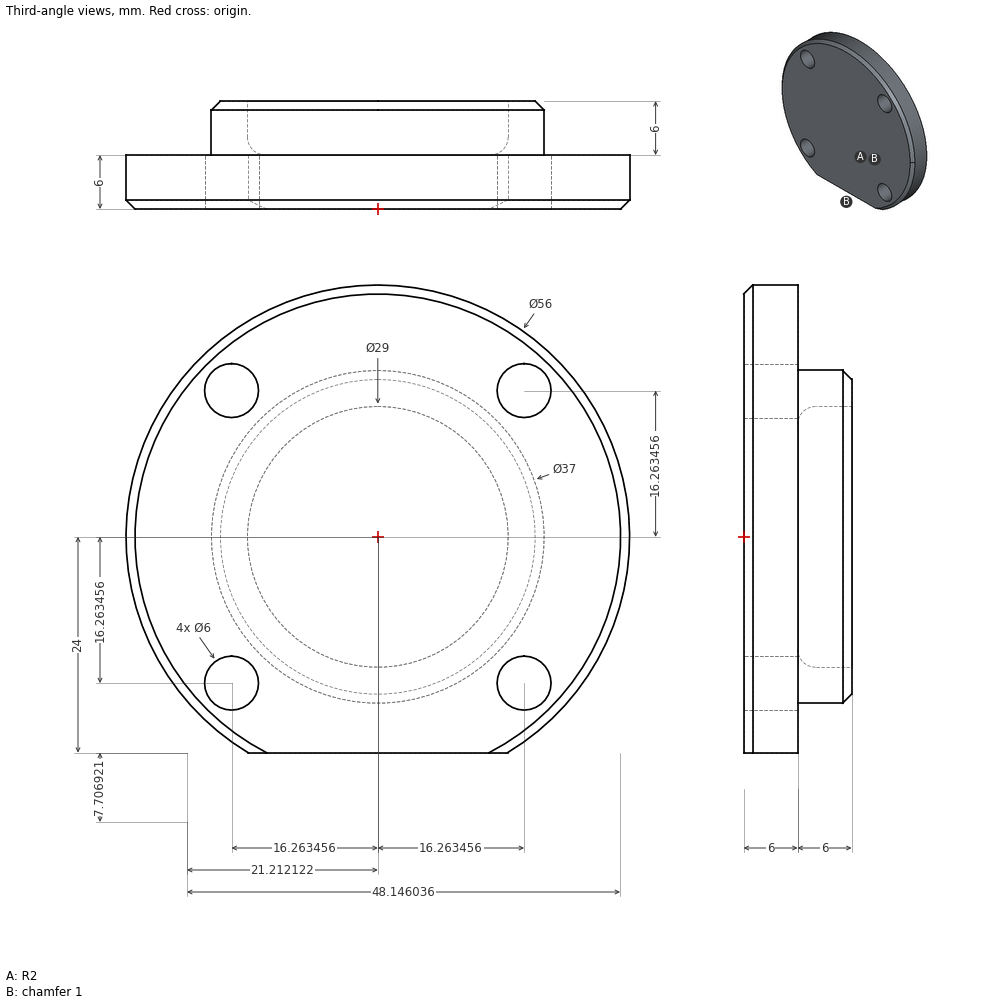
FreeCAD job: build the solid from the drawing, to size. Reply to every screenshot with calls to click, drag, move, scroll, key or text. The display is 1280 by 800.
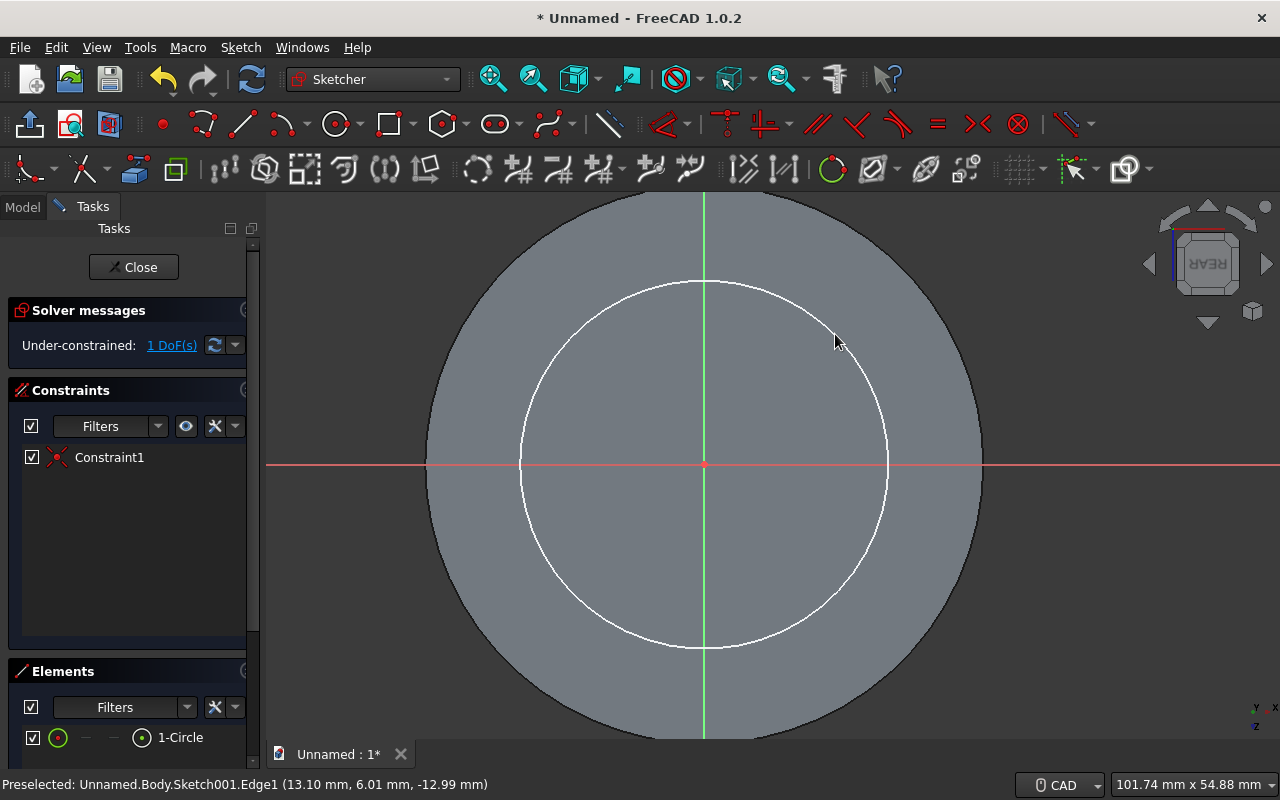
click(664, 124)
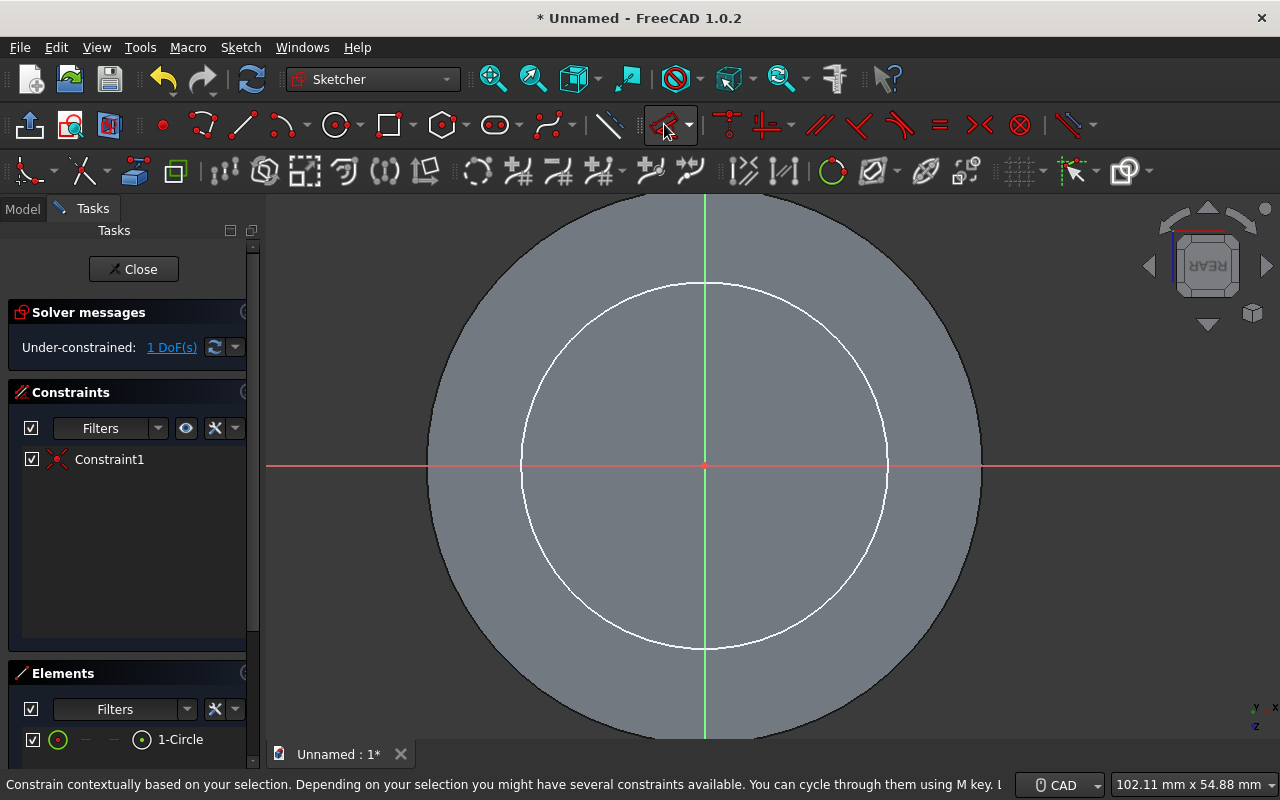
click(834, 336)
click(857, 313)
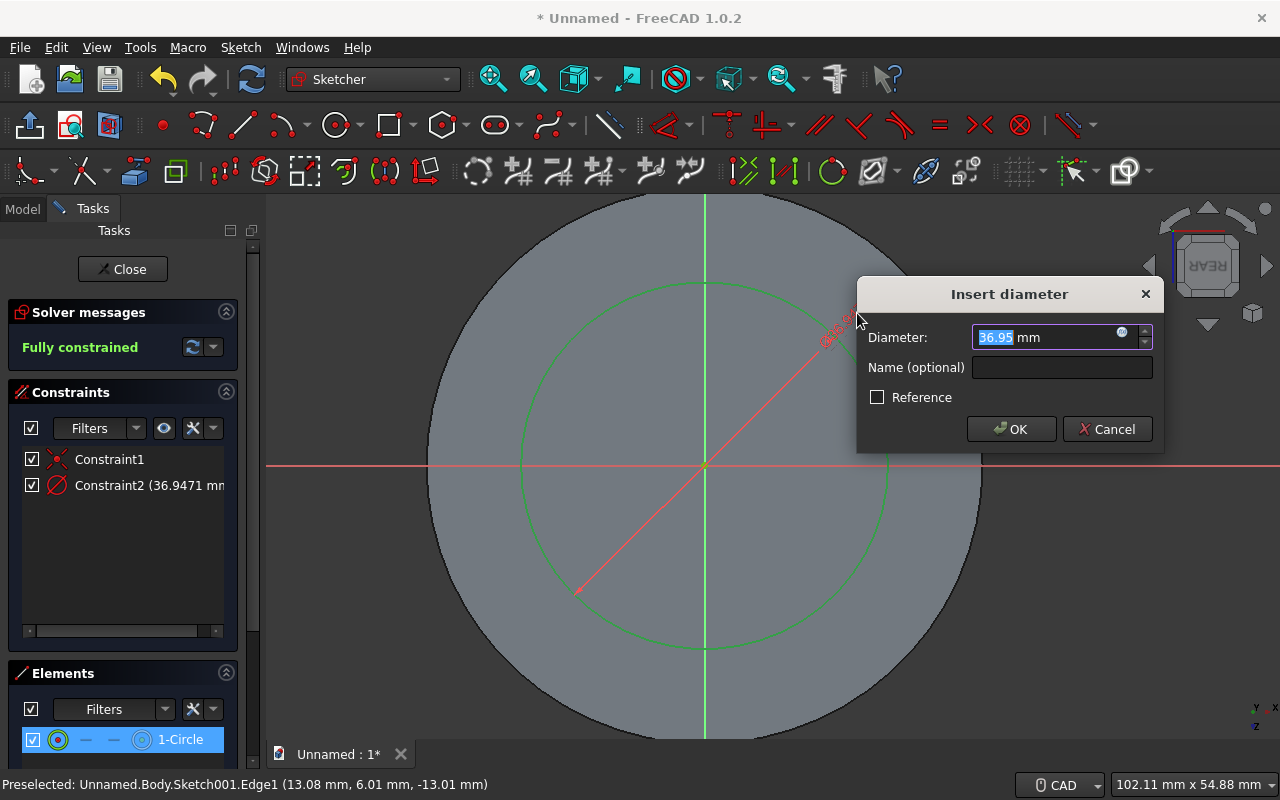
text(37)
key(Return)
key(Escape)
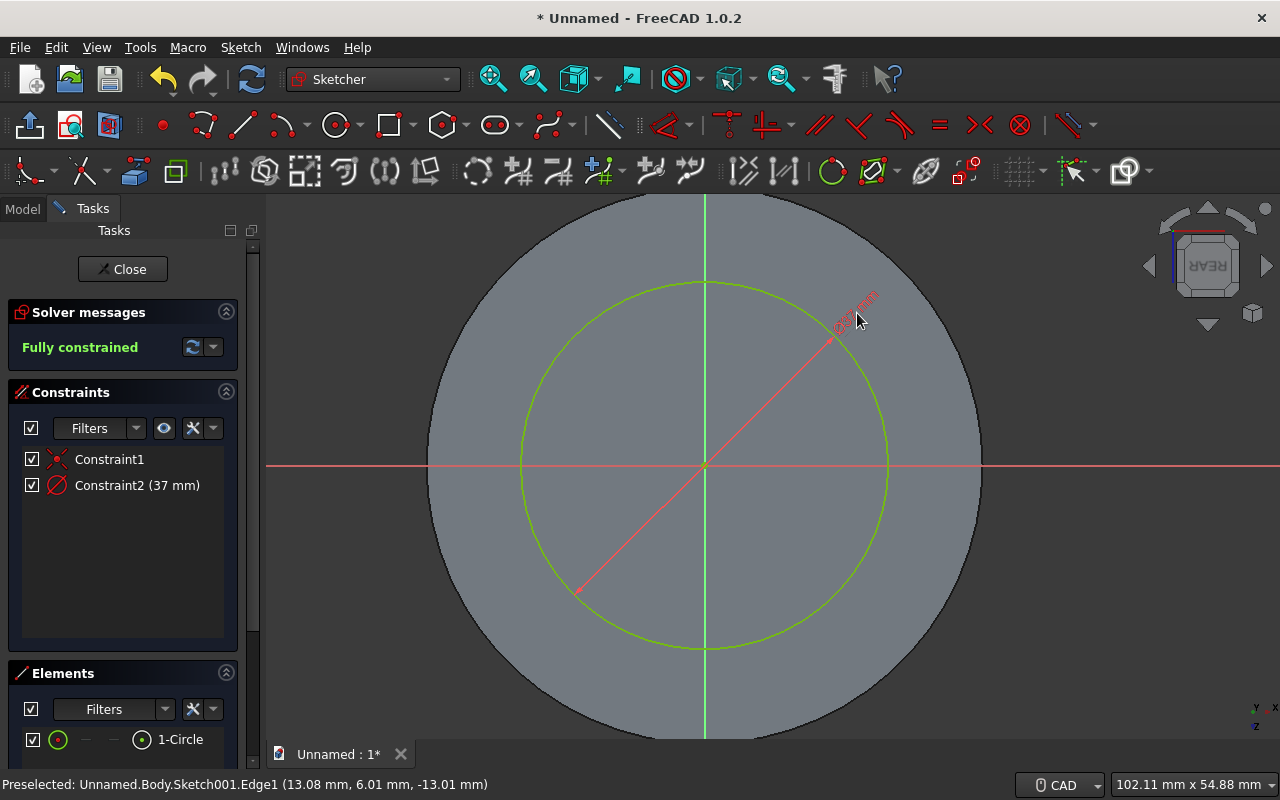
click(123, 269)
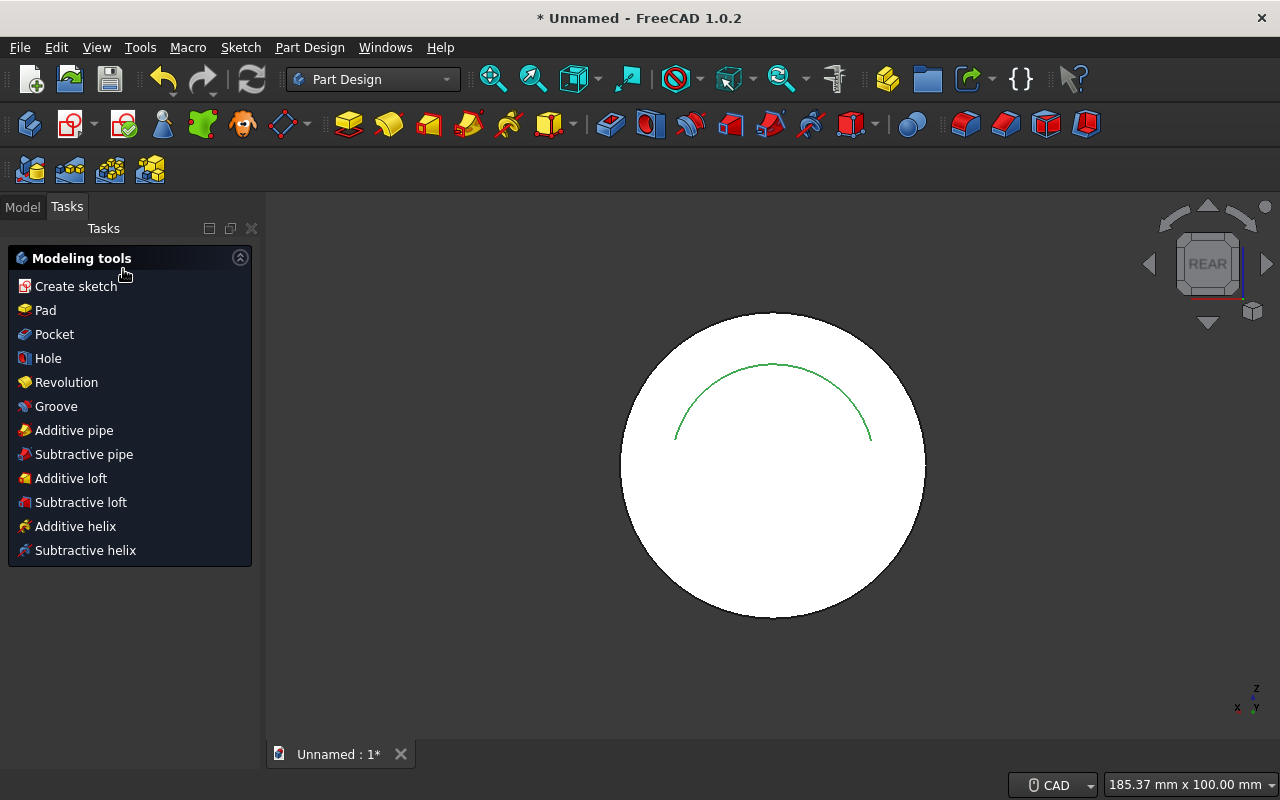
click(350, 124)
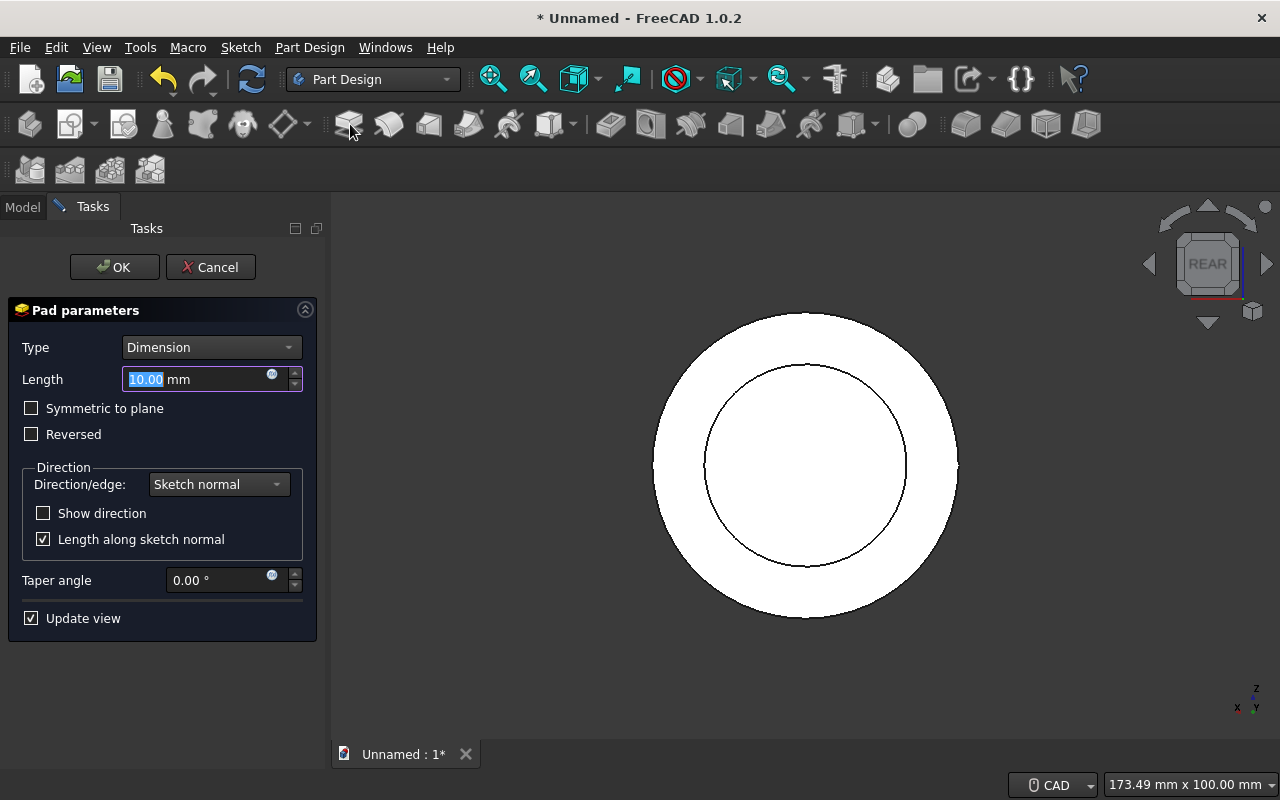
text(6)
key(Tab)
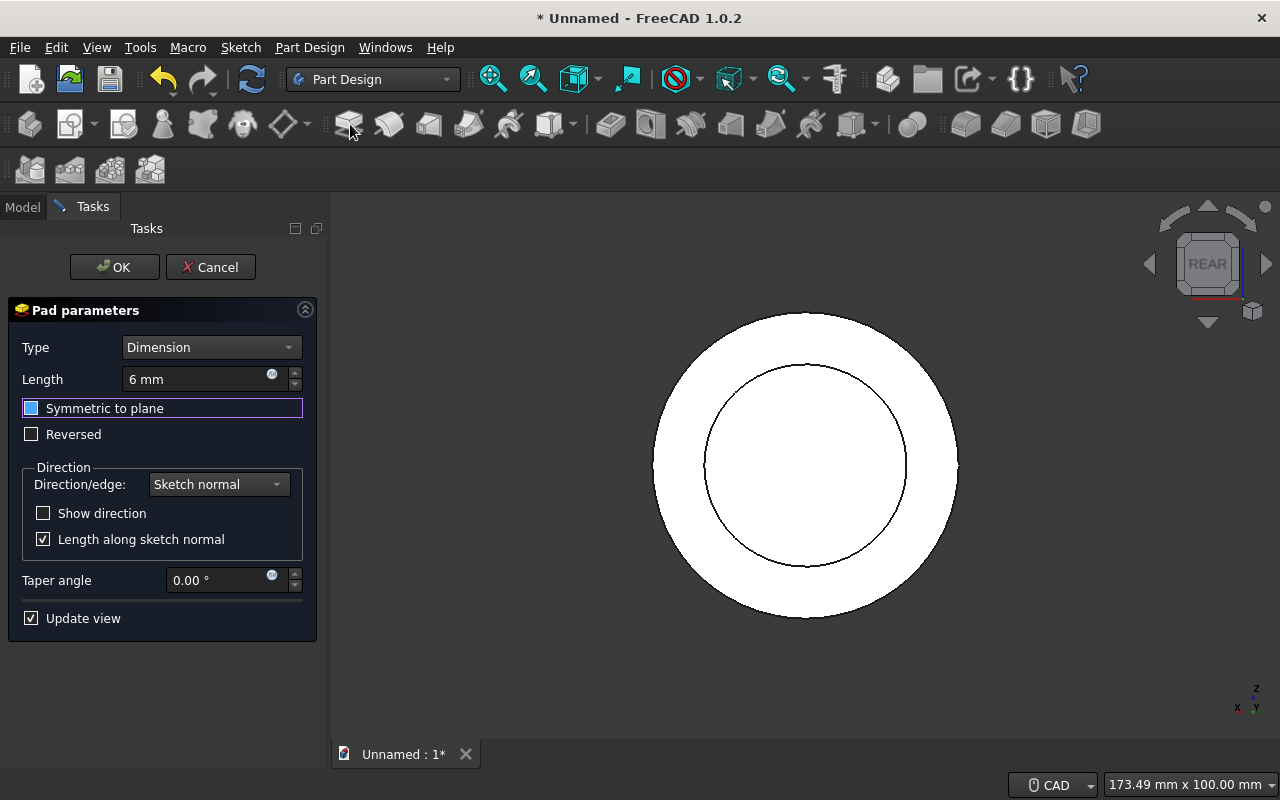
click(115, 267)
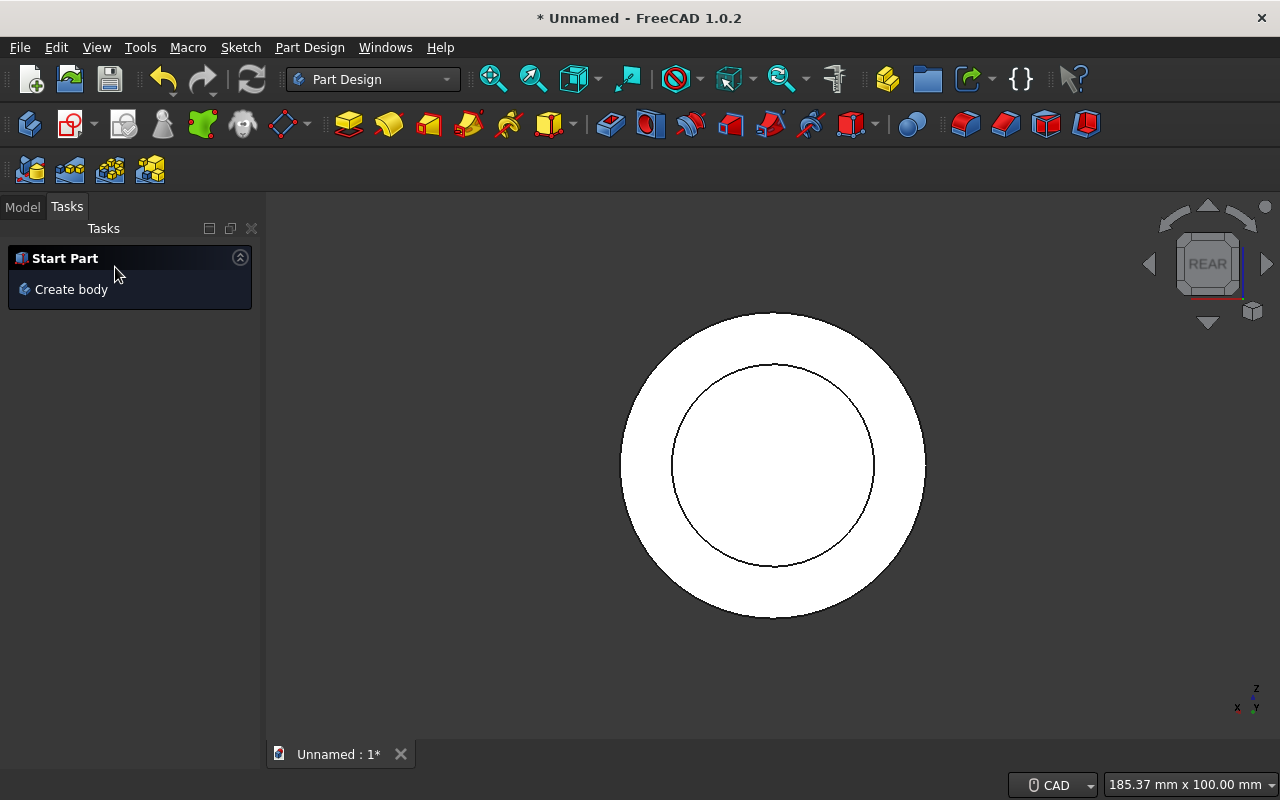
click(773, 464)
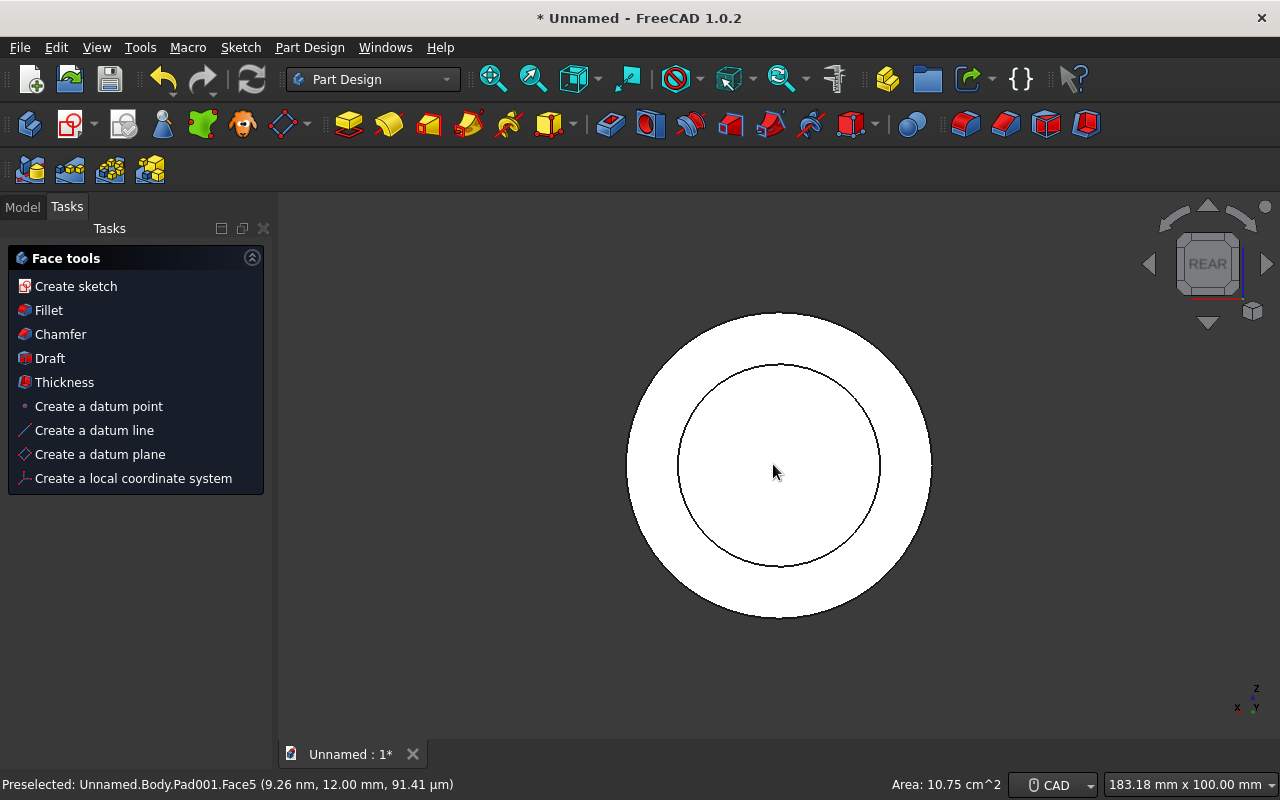
click(70, 124)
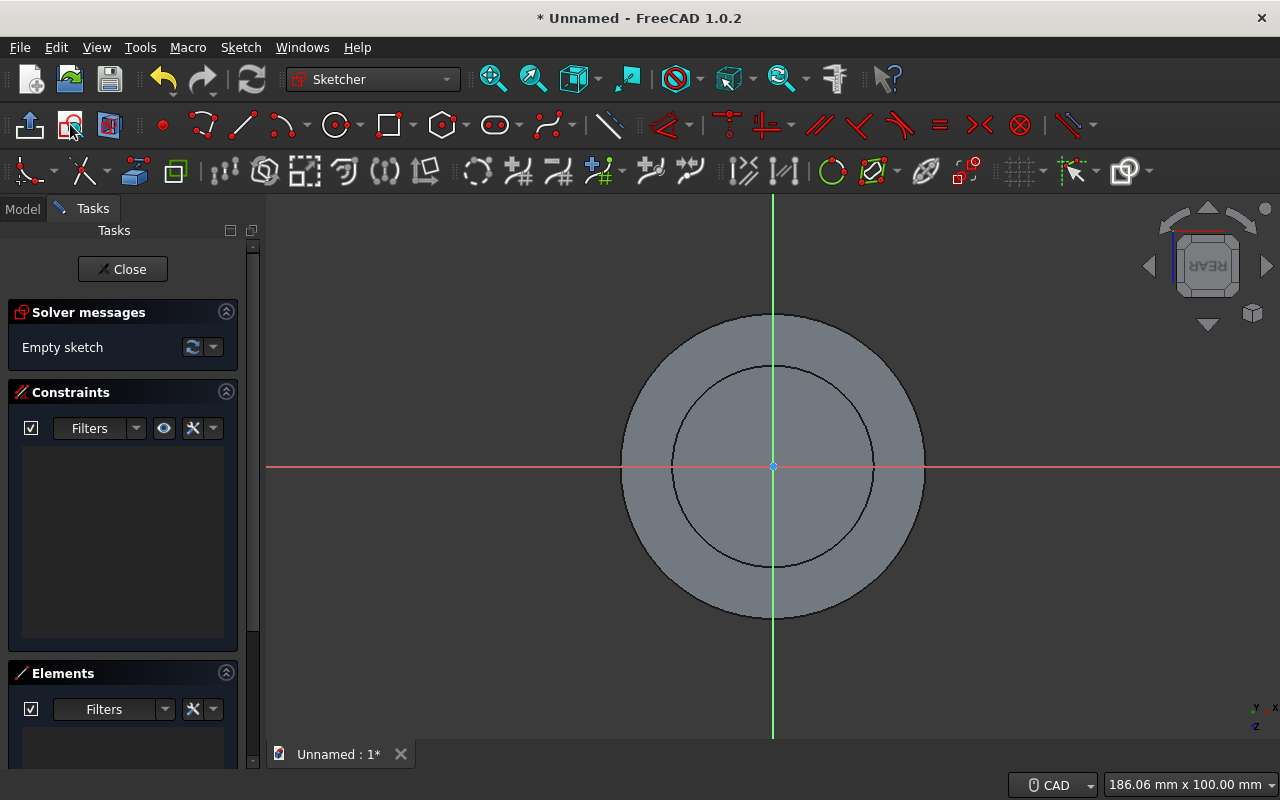
scroll(829, 466, up, 4)